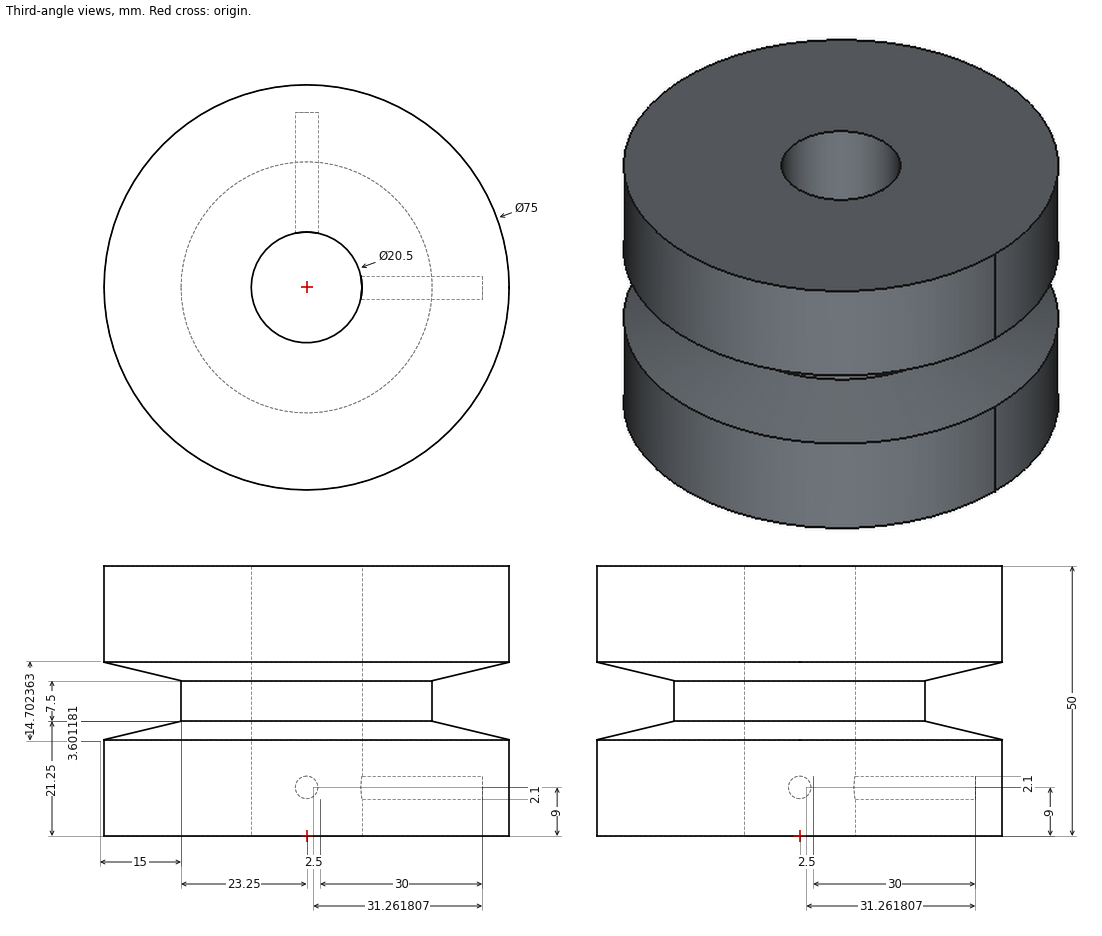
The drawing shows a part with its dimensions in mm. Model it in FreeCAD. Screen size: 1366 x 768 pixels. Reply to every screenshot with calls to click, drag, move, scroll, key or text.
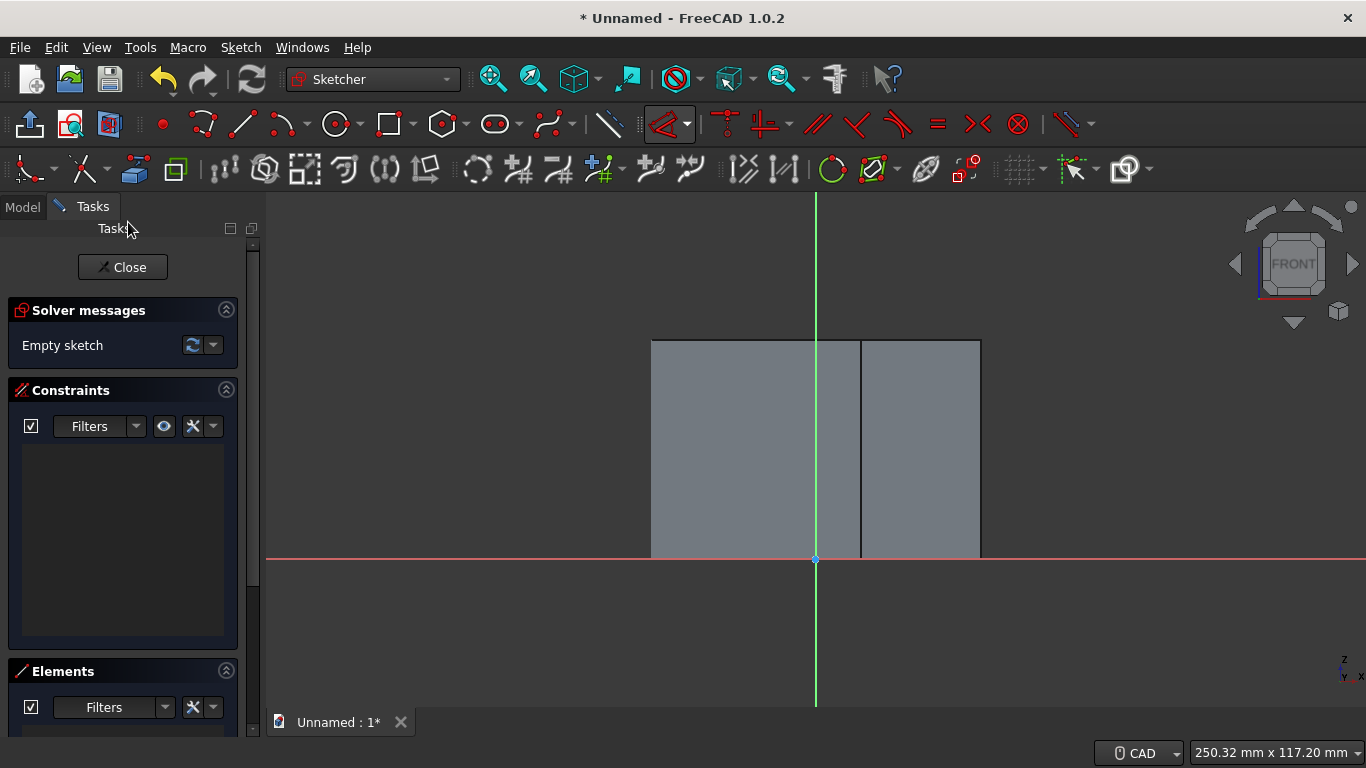
scroll(664, 450, up, 8)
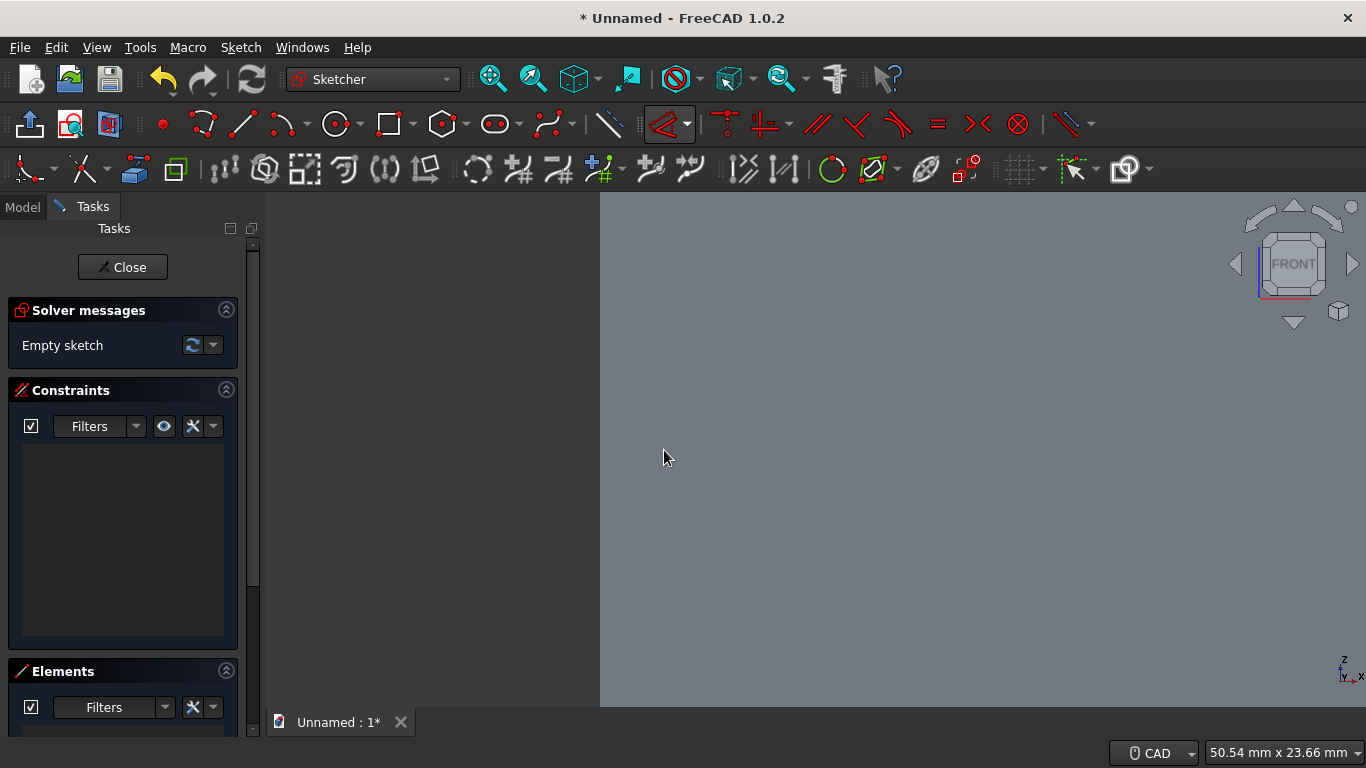
key(g)
key(m)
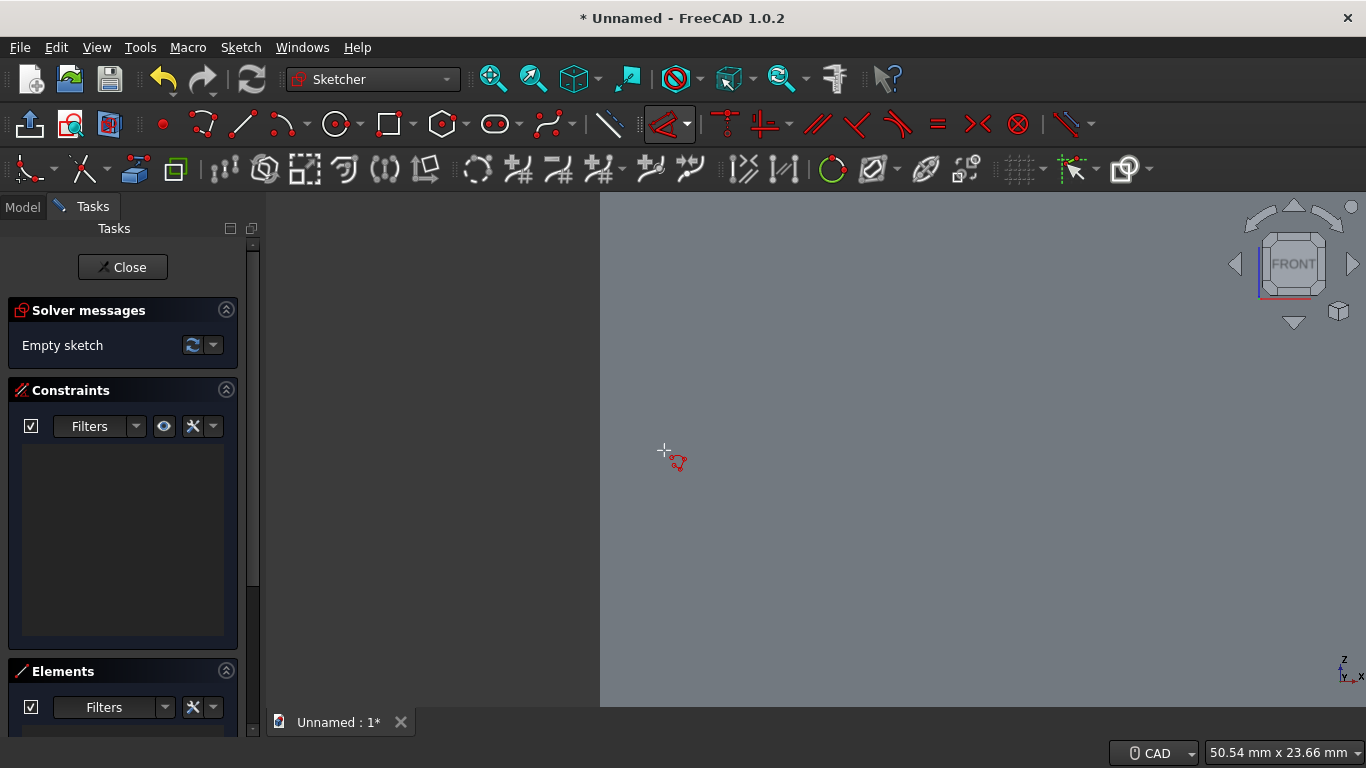
click(909, 527)
click(582, 606)
click(582, 286)
click(909, 364)
click(909, 528)
key(Escape)
key(Escape)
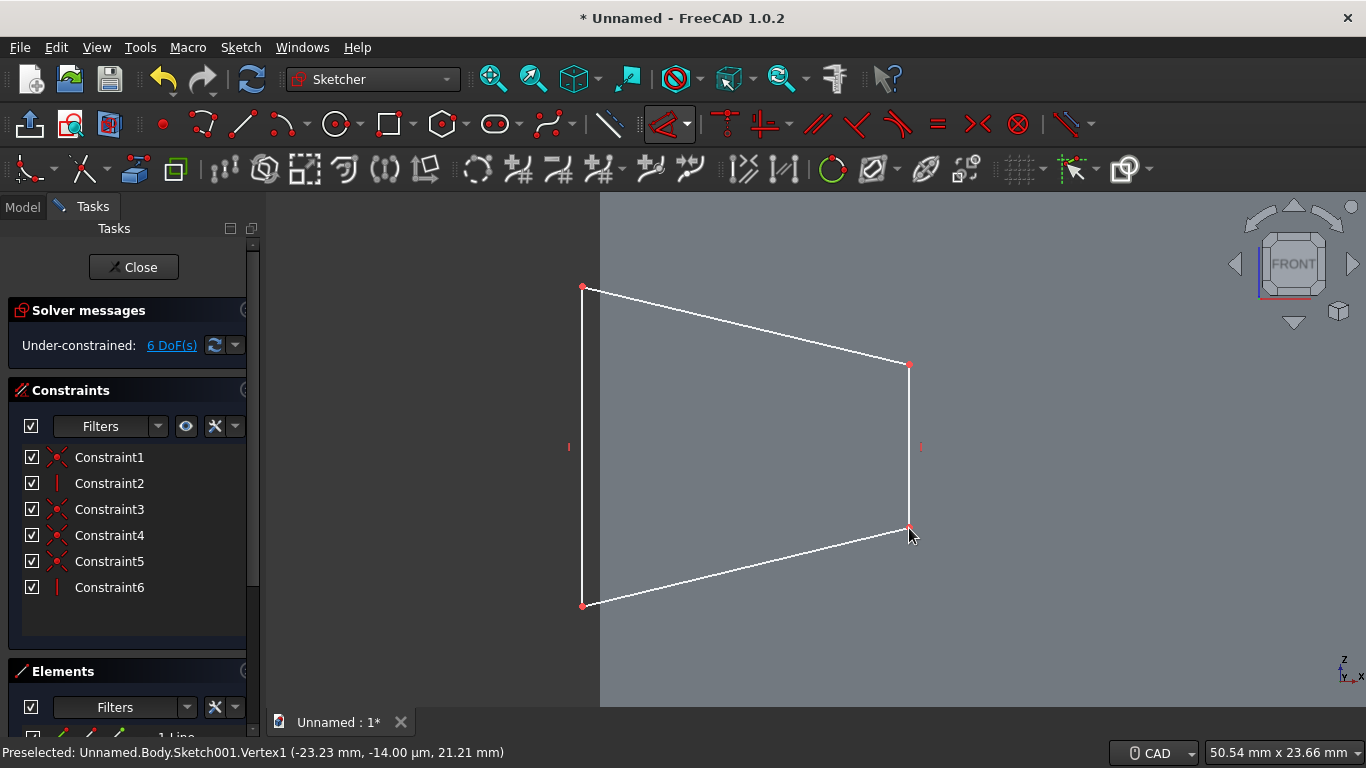
key(d)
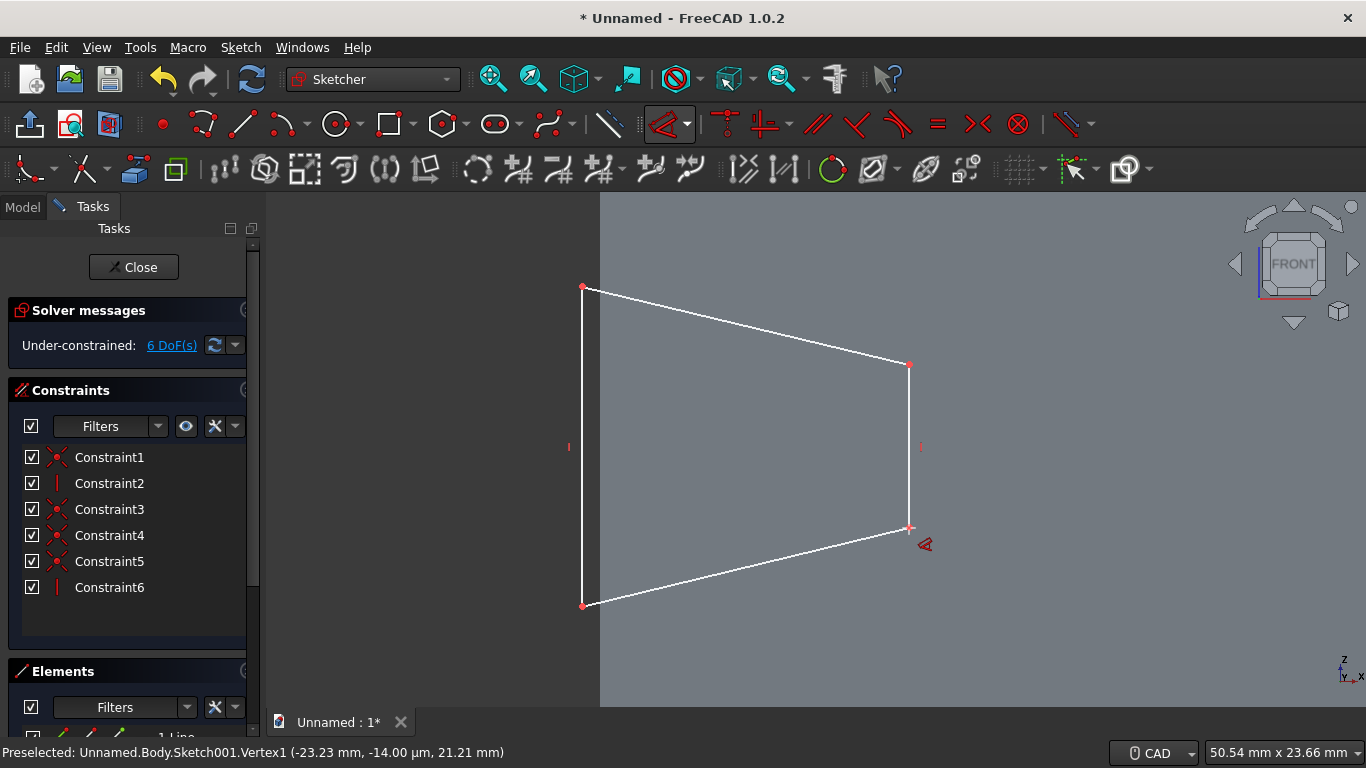
click(909, 414)
click(943, 447)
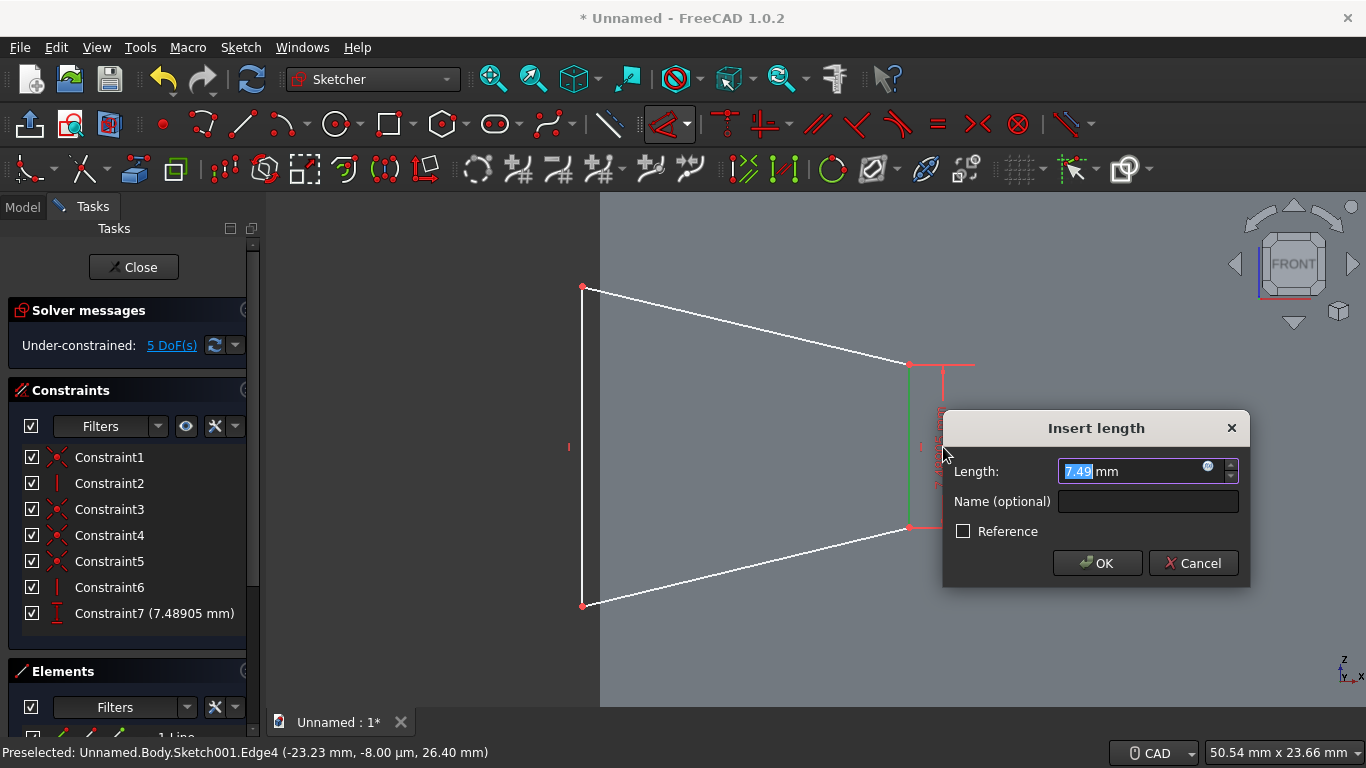
text(7.5)
key(Return)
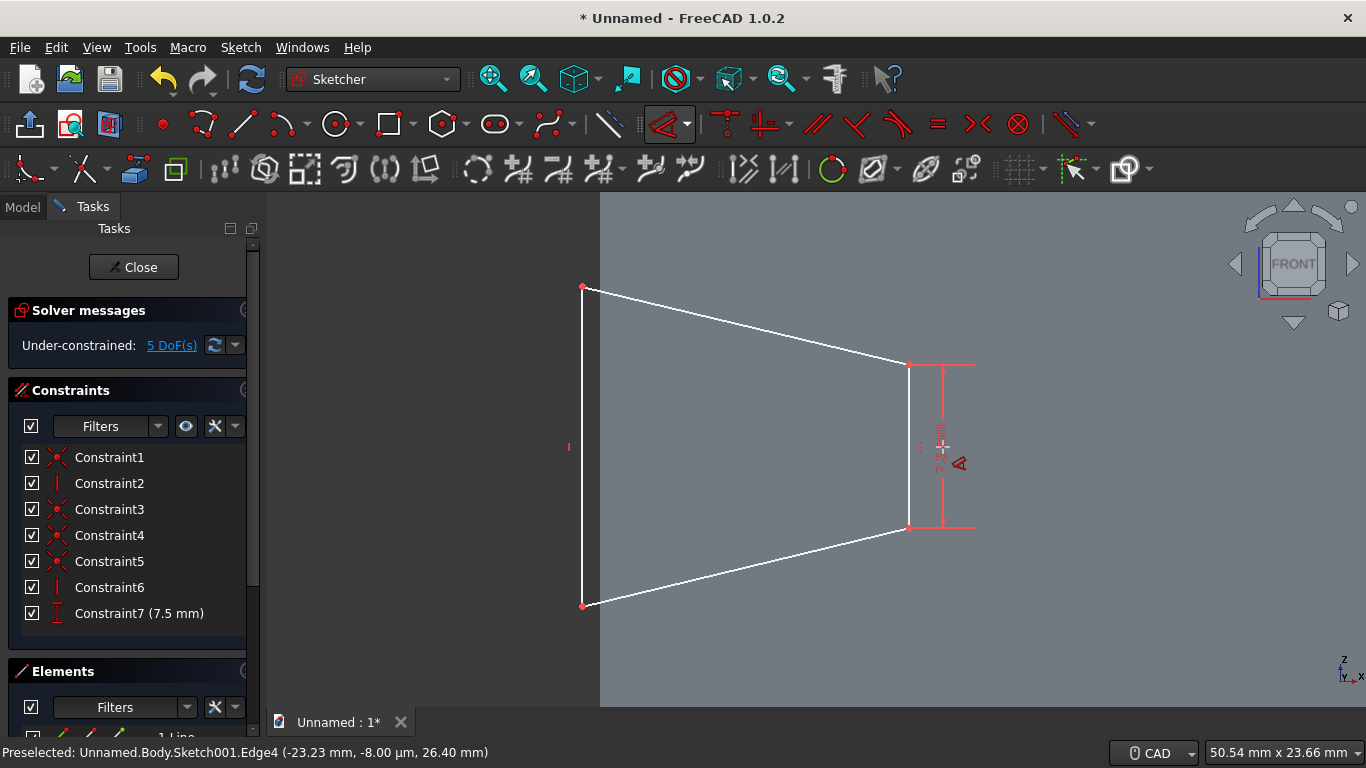
click(811, 552)
click(745, 641)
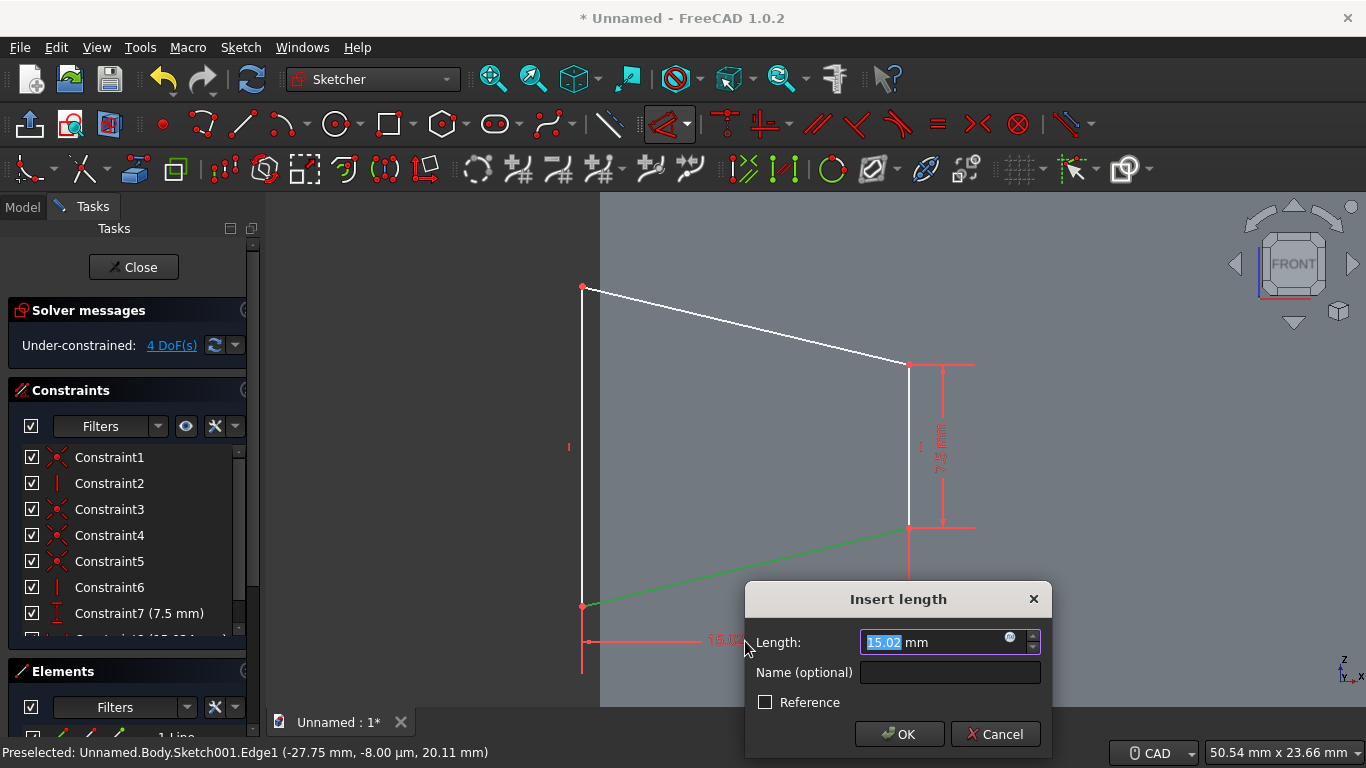
text(15)
key(Return)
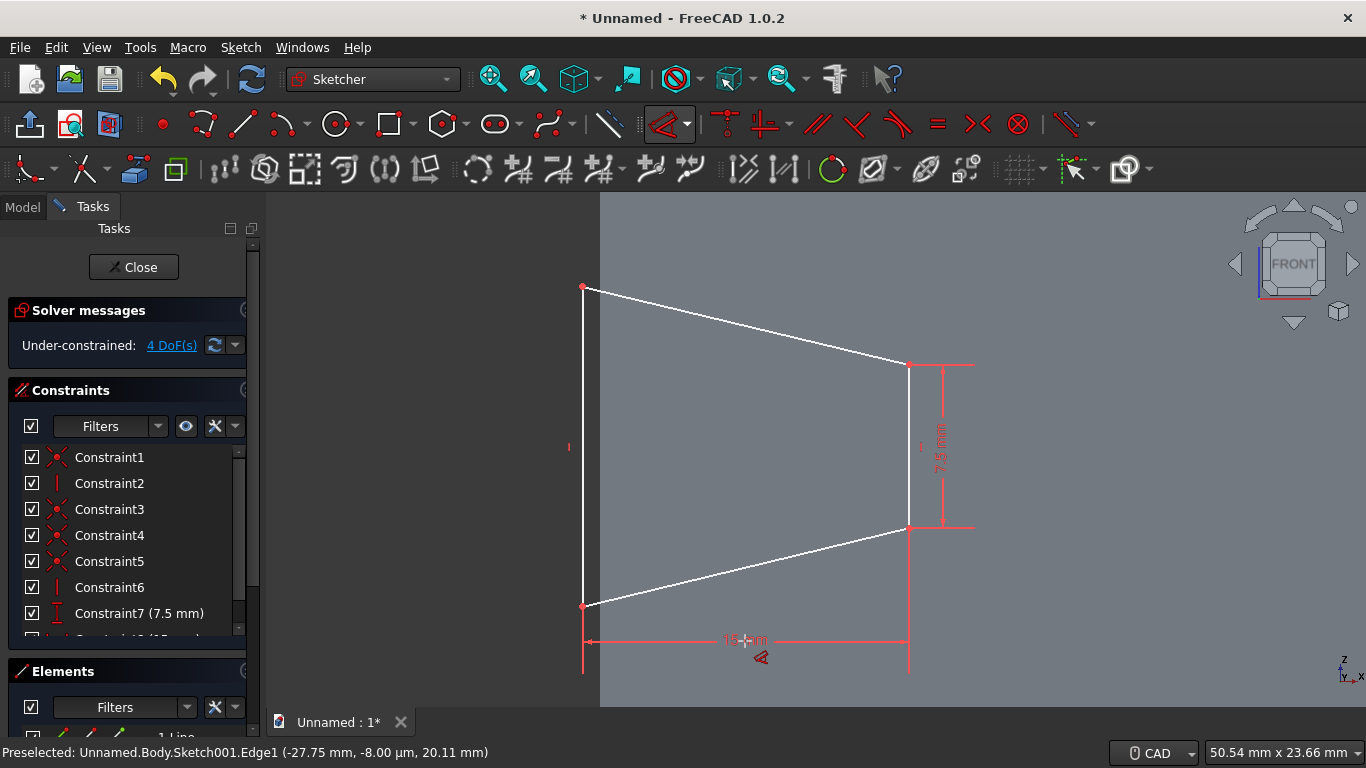
click(909, 528)
click(1055, 494)